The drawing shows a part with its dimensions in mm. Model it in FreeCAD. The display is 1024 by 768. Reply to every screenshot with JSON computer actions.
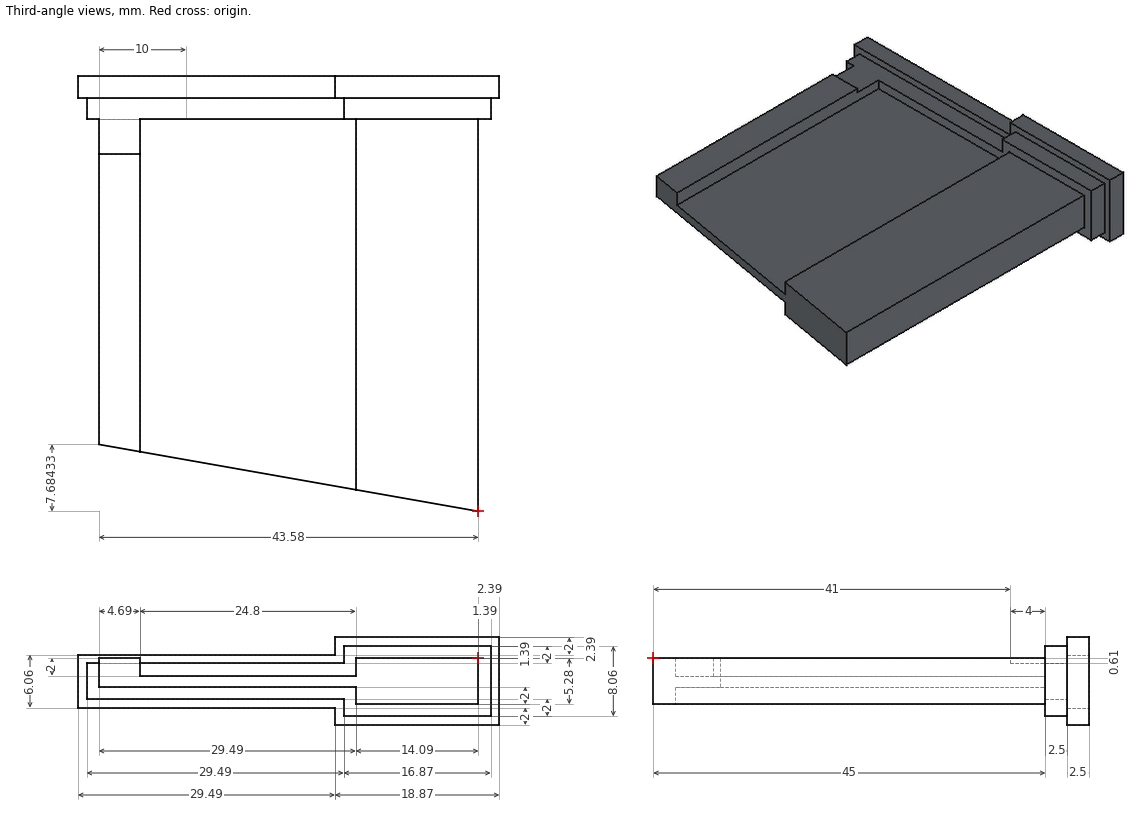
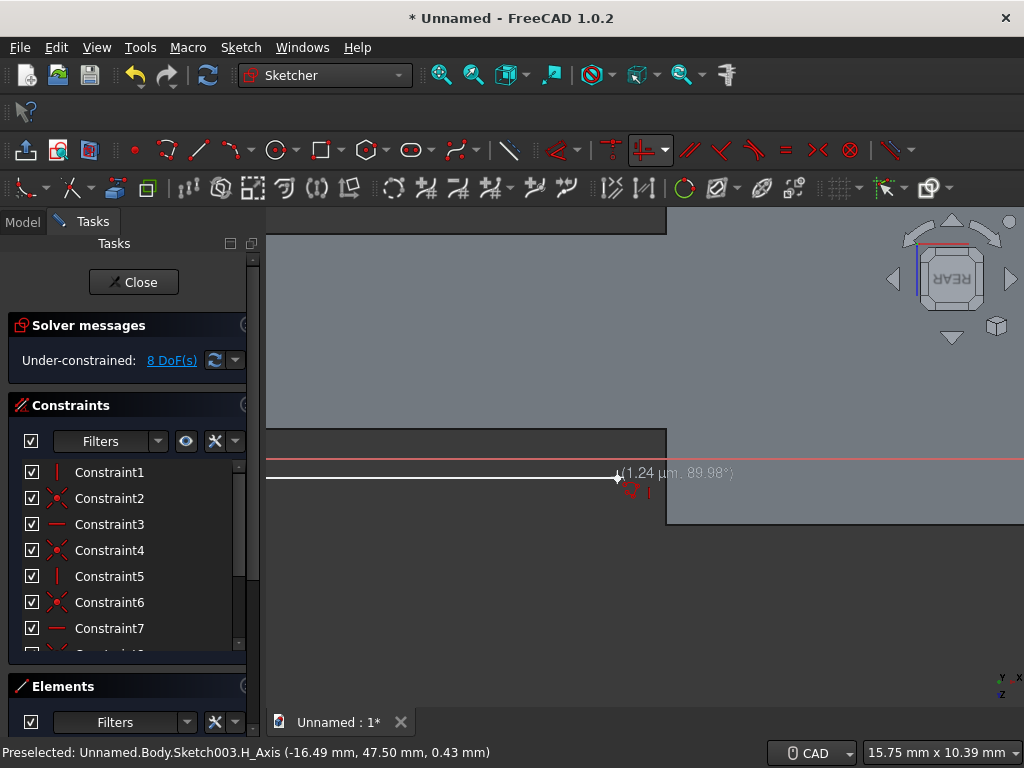
{"action": "scroll", "coordinate": [619, 482], "scroll_direction": "down", "scroll_amount": 9}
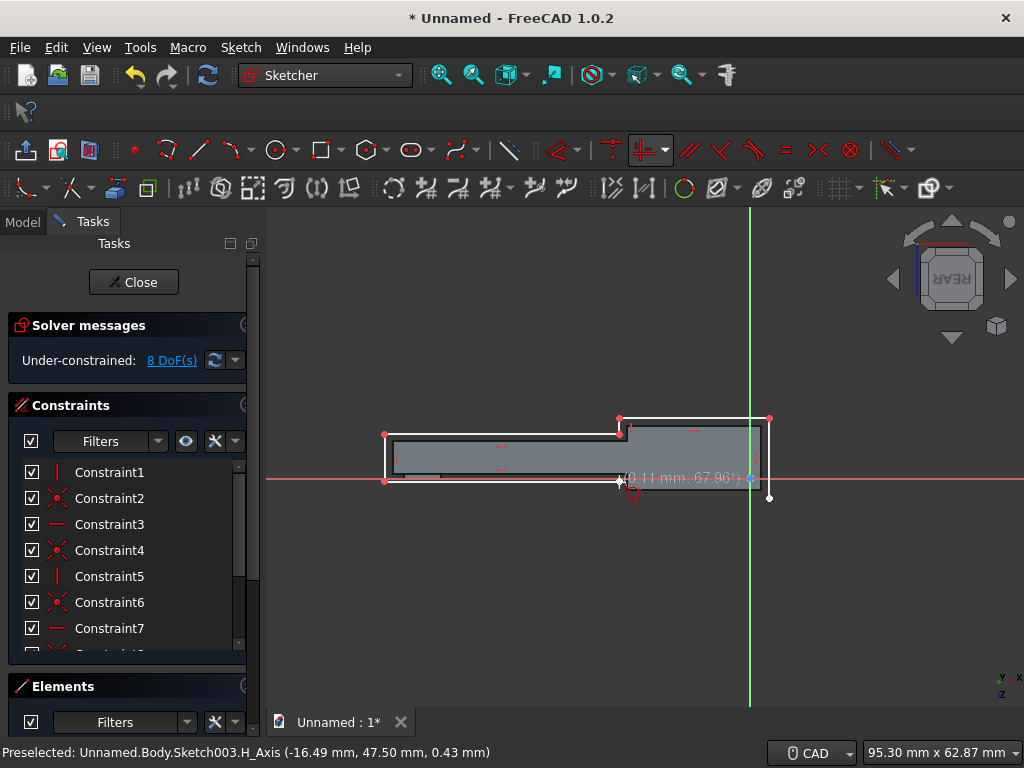
{"action": "left_click", "coordinate": [619, 498]}
{"action": "left_click", "coordinate": [769, 499]}
{"action": "key", "text": "Escape"}
{"action": "key", "text": "Escape"}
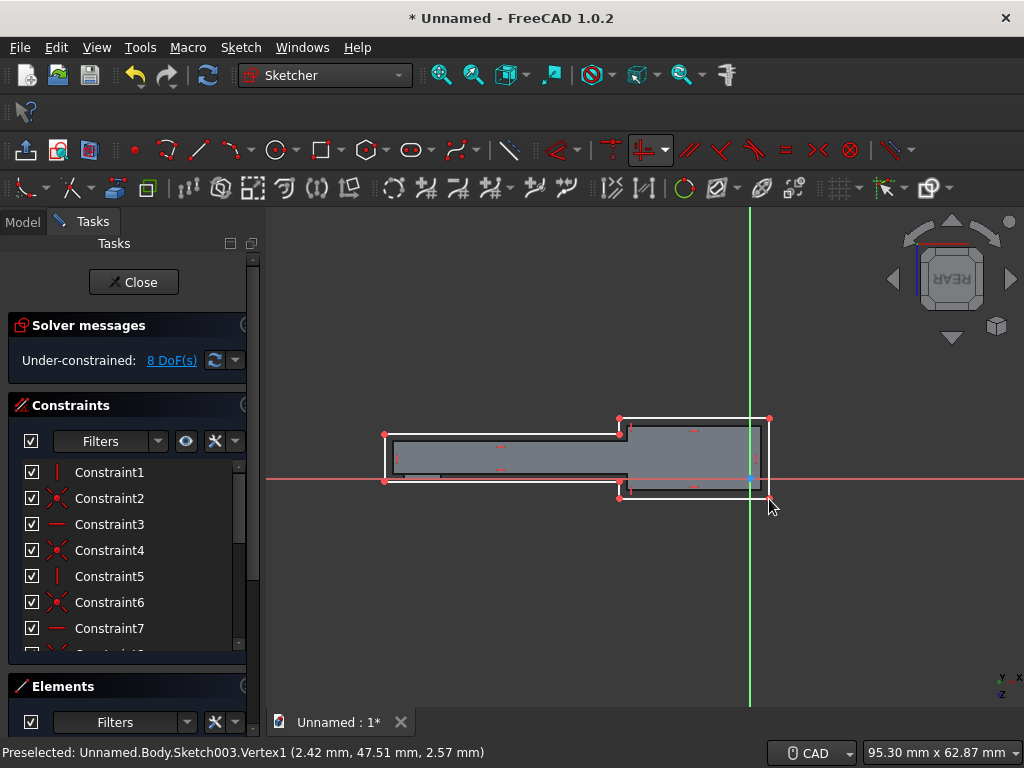
{"action": "key", "text": "d"}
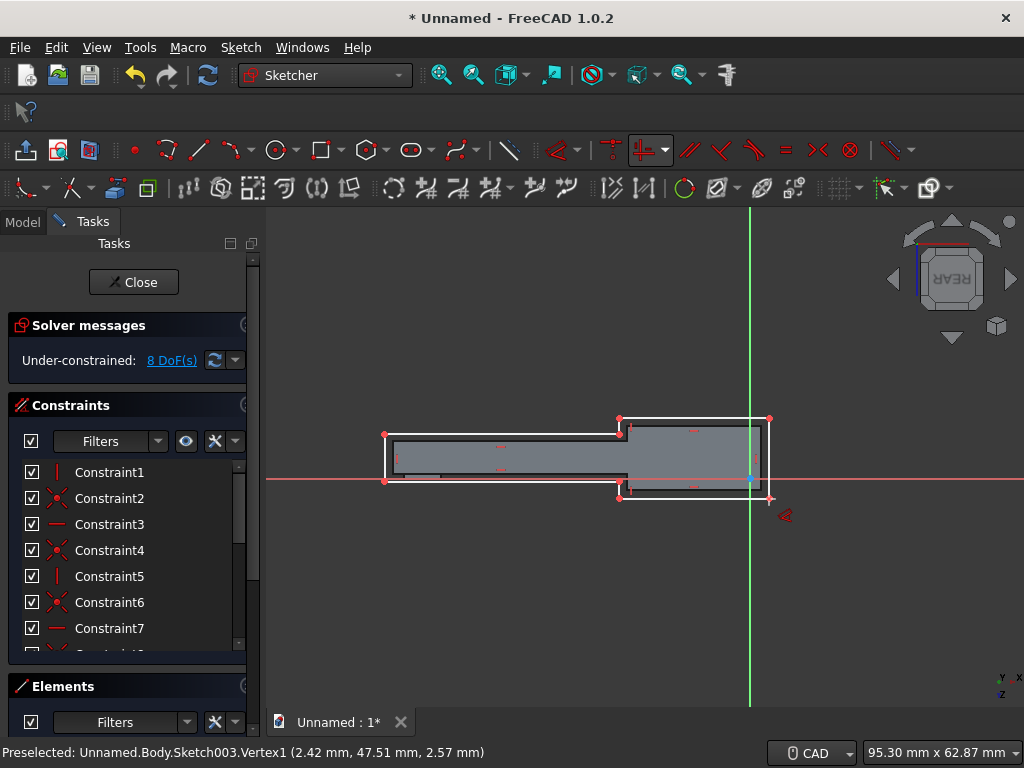
{"action": "scroll", "coordinate": [619, 426], "scroll_direction": "up", "scroll_amount": 5}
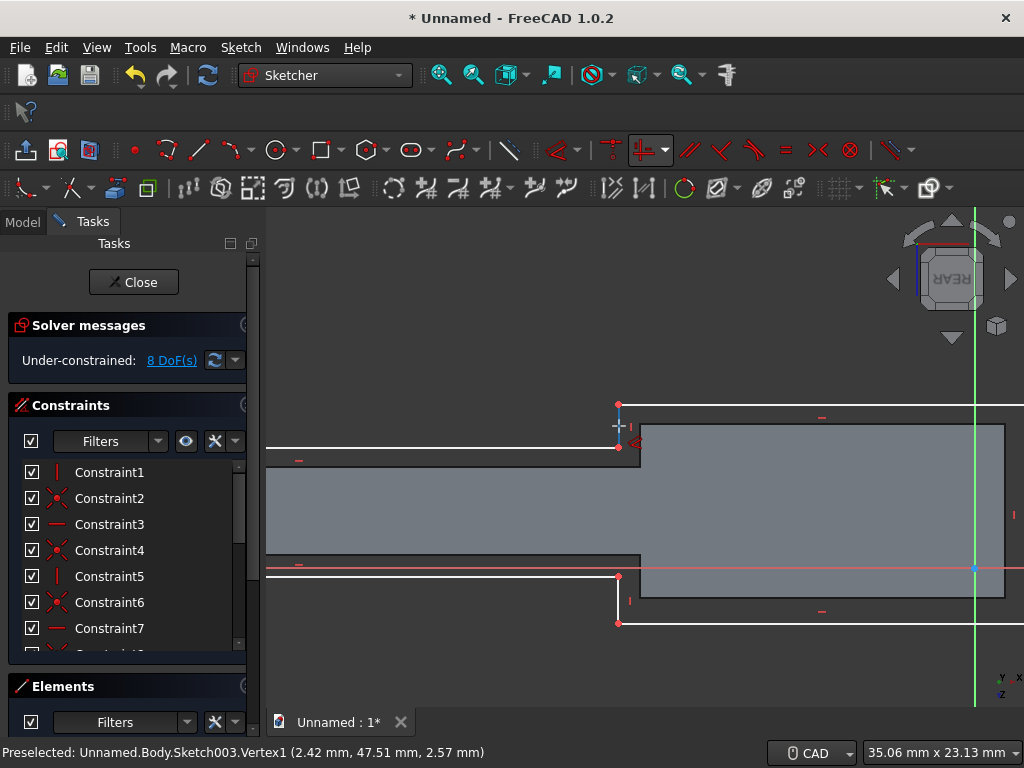
{"action": "left_click", "coordinate": [619, 426]}
{"action": "left_click", "coordinate": [653, 426]}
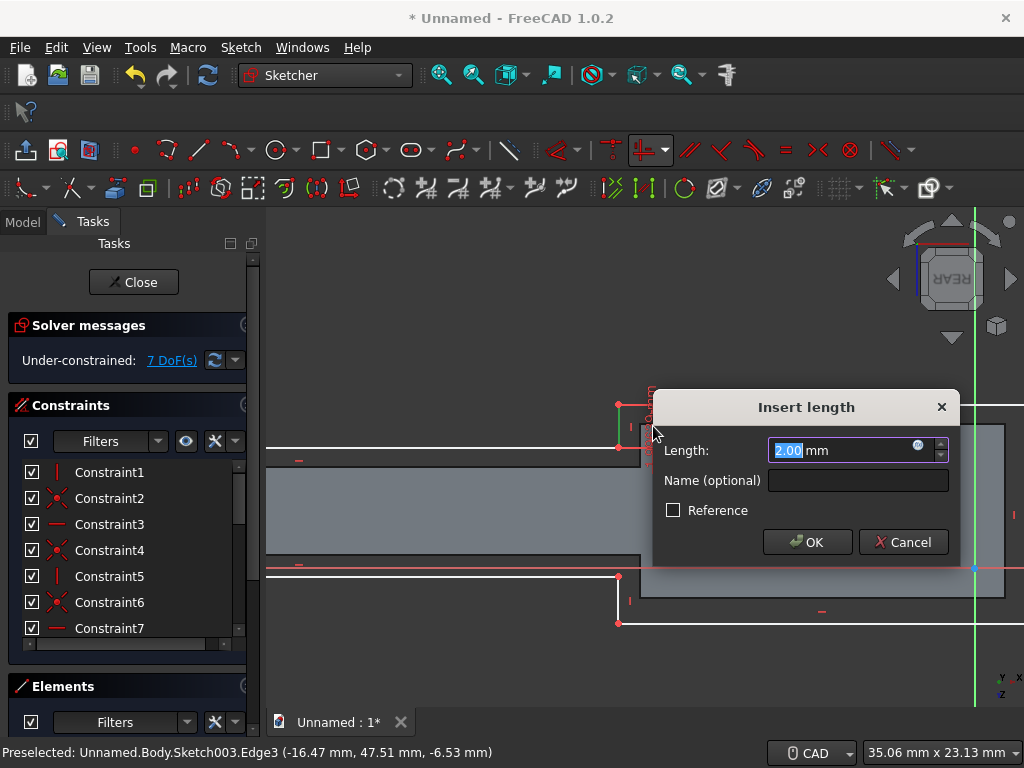
{"action": "type", "text": "2"}
{"action": "key", "text": "Return"}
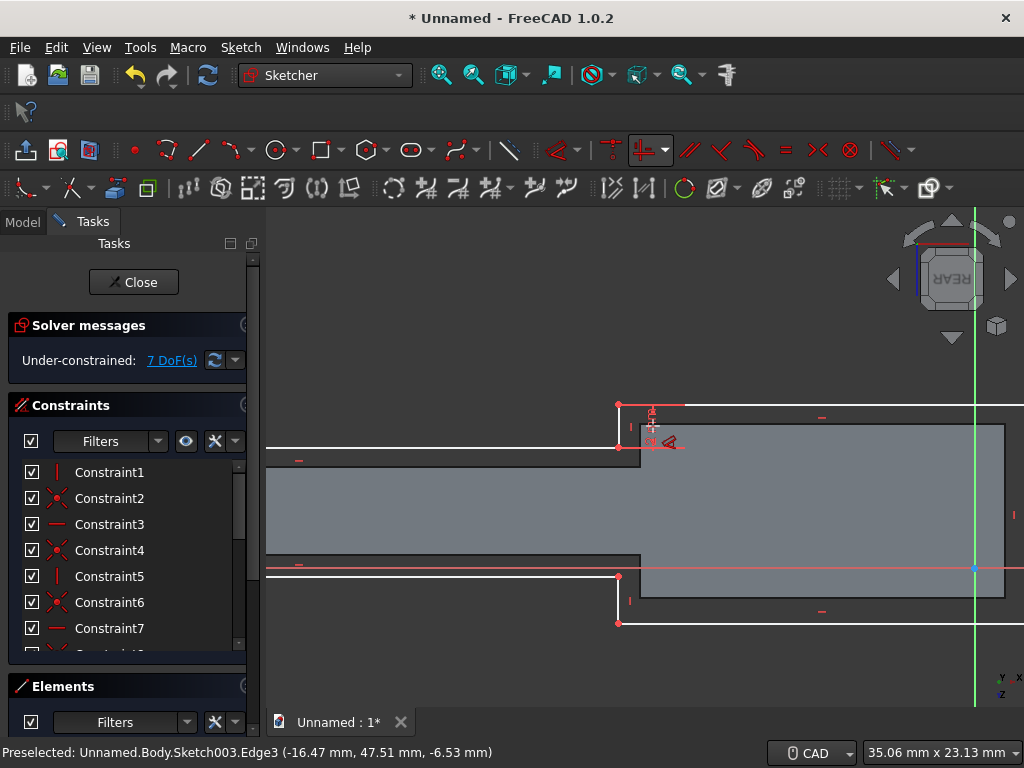
{"action": "left_click", "coordinate": [618, 591]}
{"action": "left_click", "coordinate": [652, 600]}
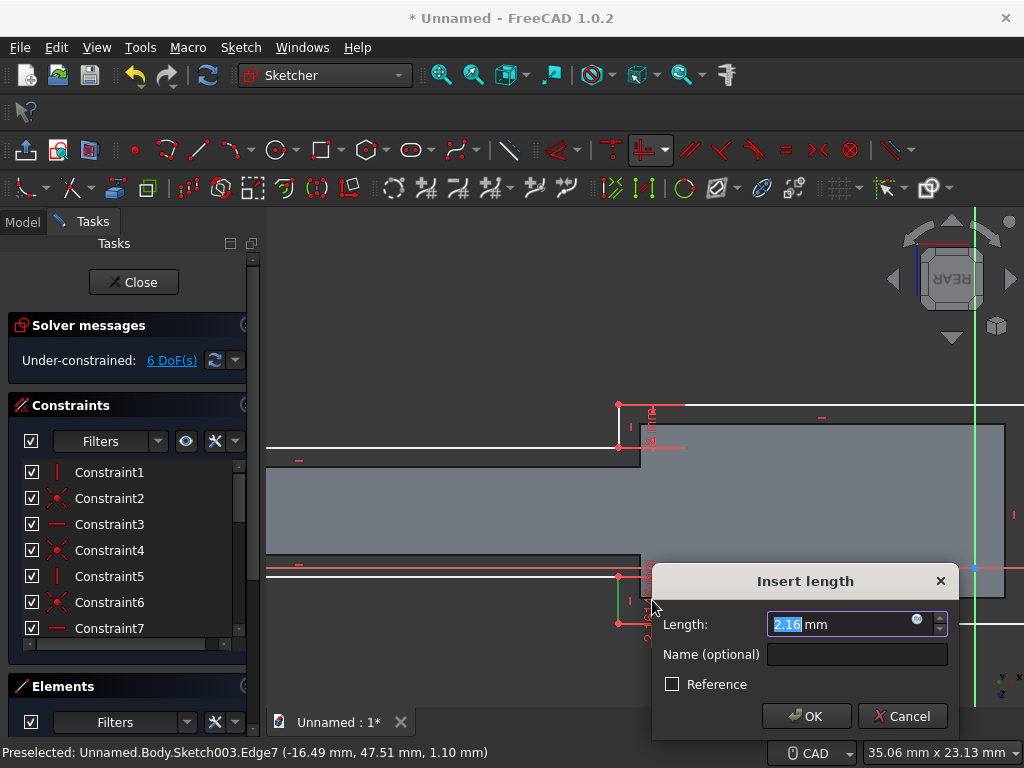
{"action": "type", "text": "2"}
{"action": "key", "text": "Return"}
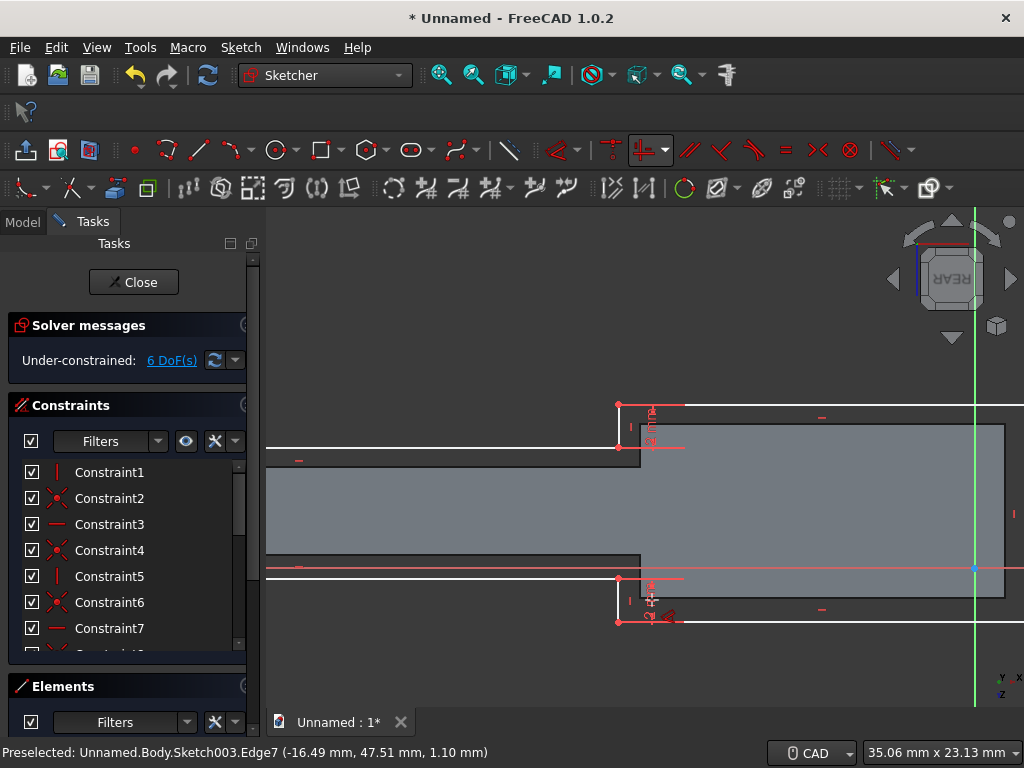
{"action": "scroll", "coordinate": [619, 426], "scroll_direction": "down", "scroll_amount": 5}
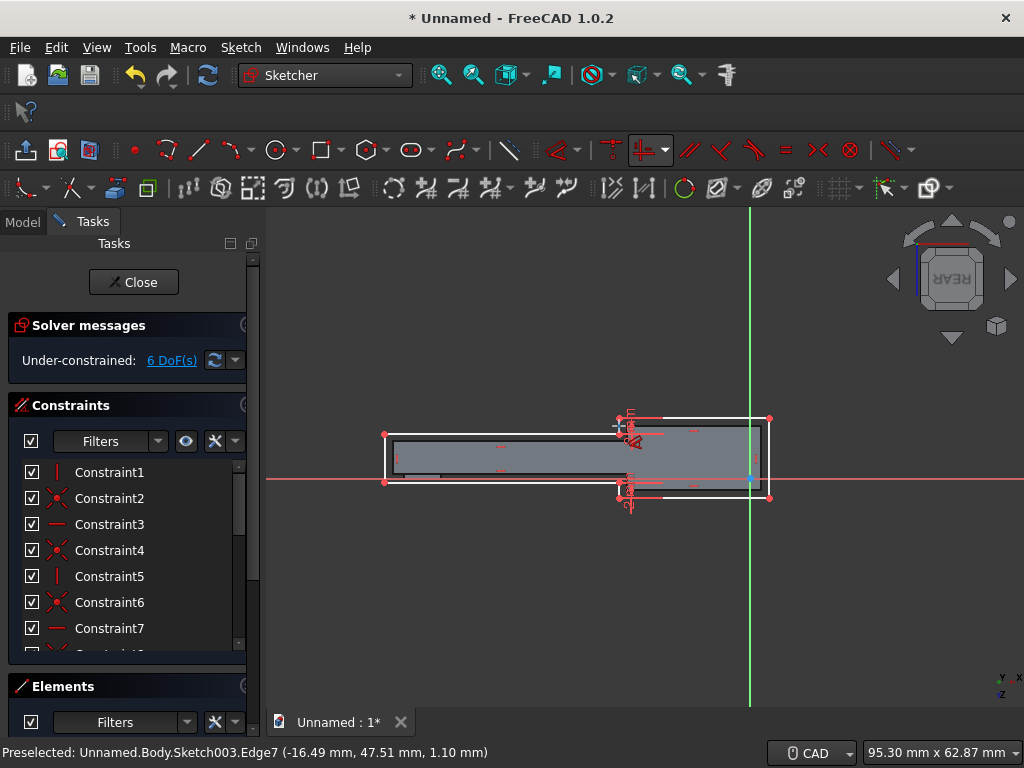
{"action": "left_click", "coordinate": [385, 449]}
{"action": "left_click", "coordinate": [351, 458]}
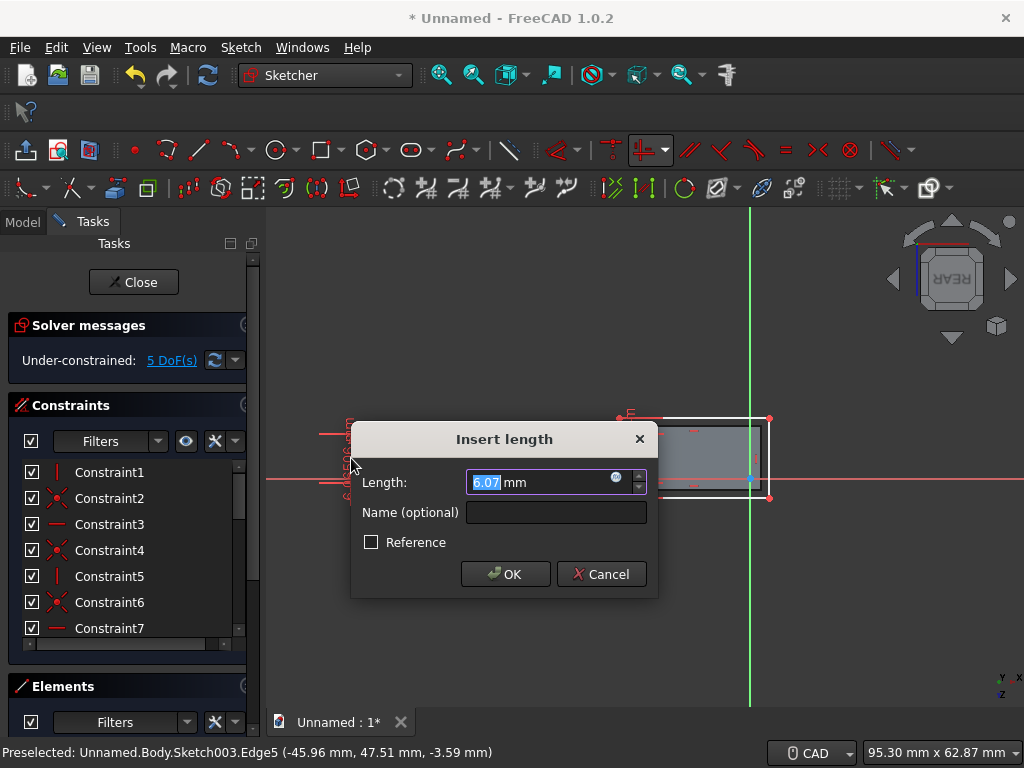
{"action": "type", "text": "6.06"}
{"action": "key", "text": "Return"}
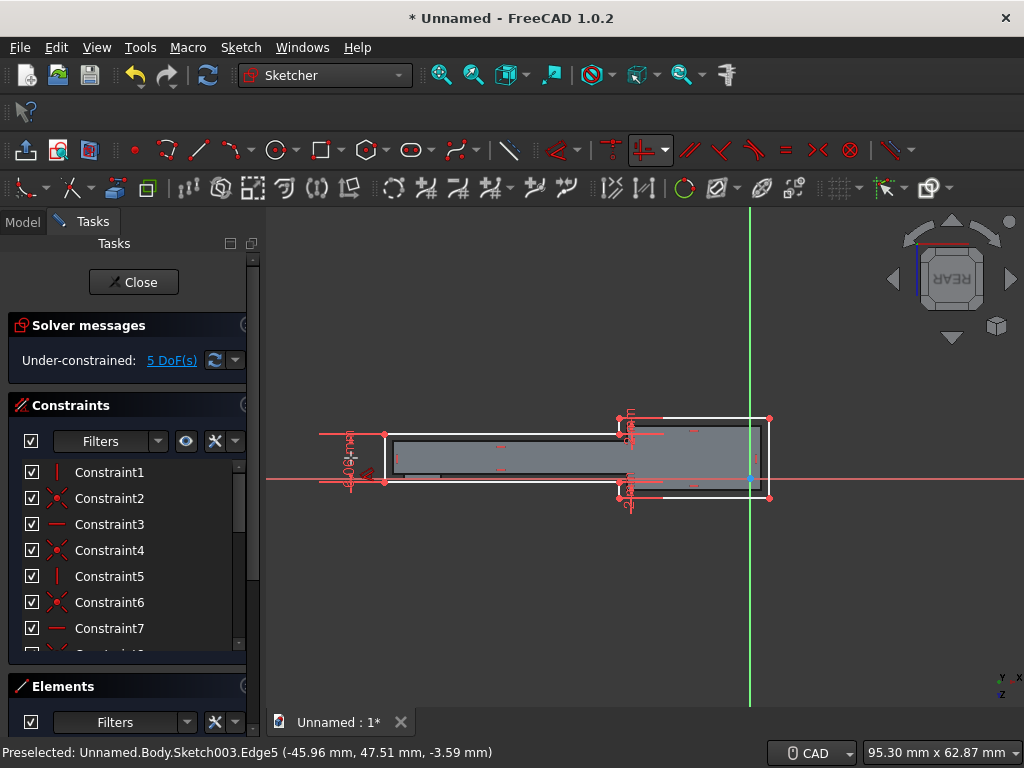
{"action": "left_click", "coordinate": [724, 418]}
{"action": "left_click", "coordinate": [694, 384]}